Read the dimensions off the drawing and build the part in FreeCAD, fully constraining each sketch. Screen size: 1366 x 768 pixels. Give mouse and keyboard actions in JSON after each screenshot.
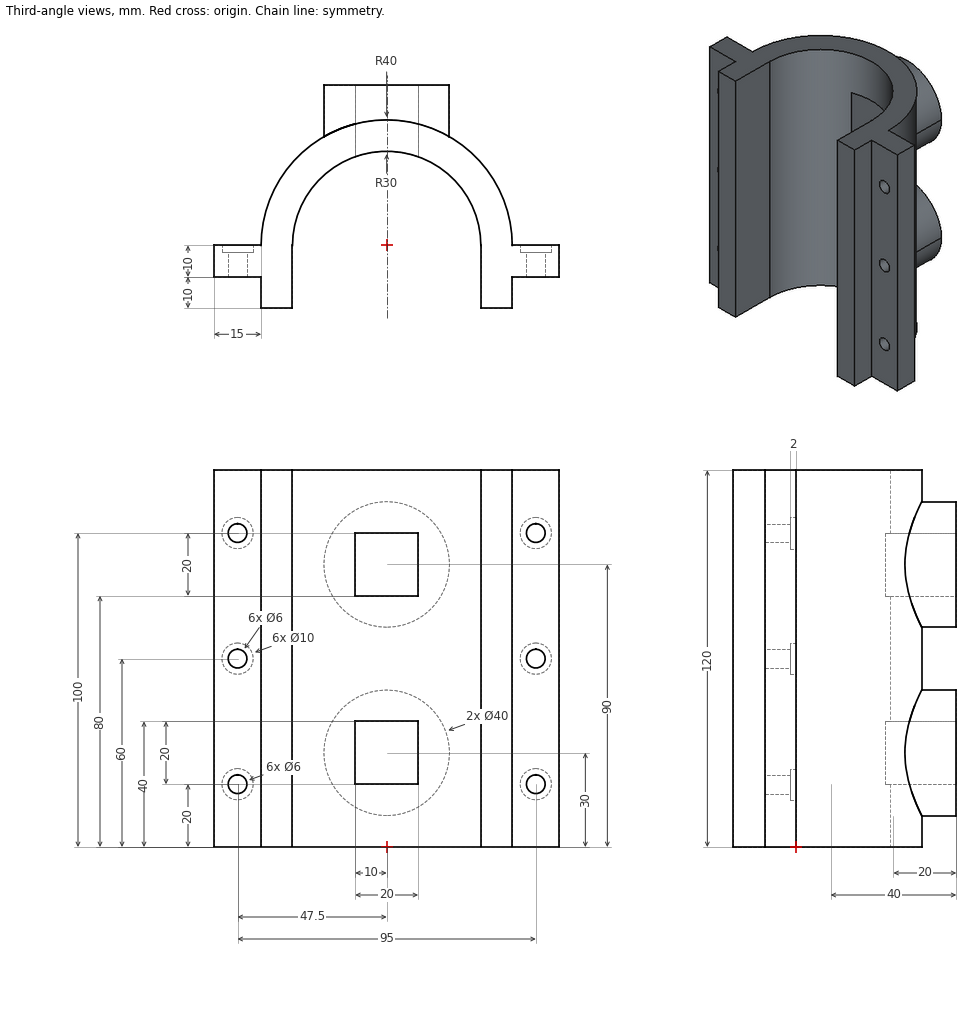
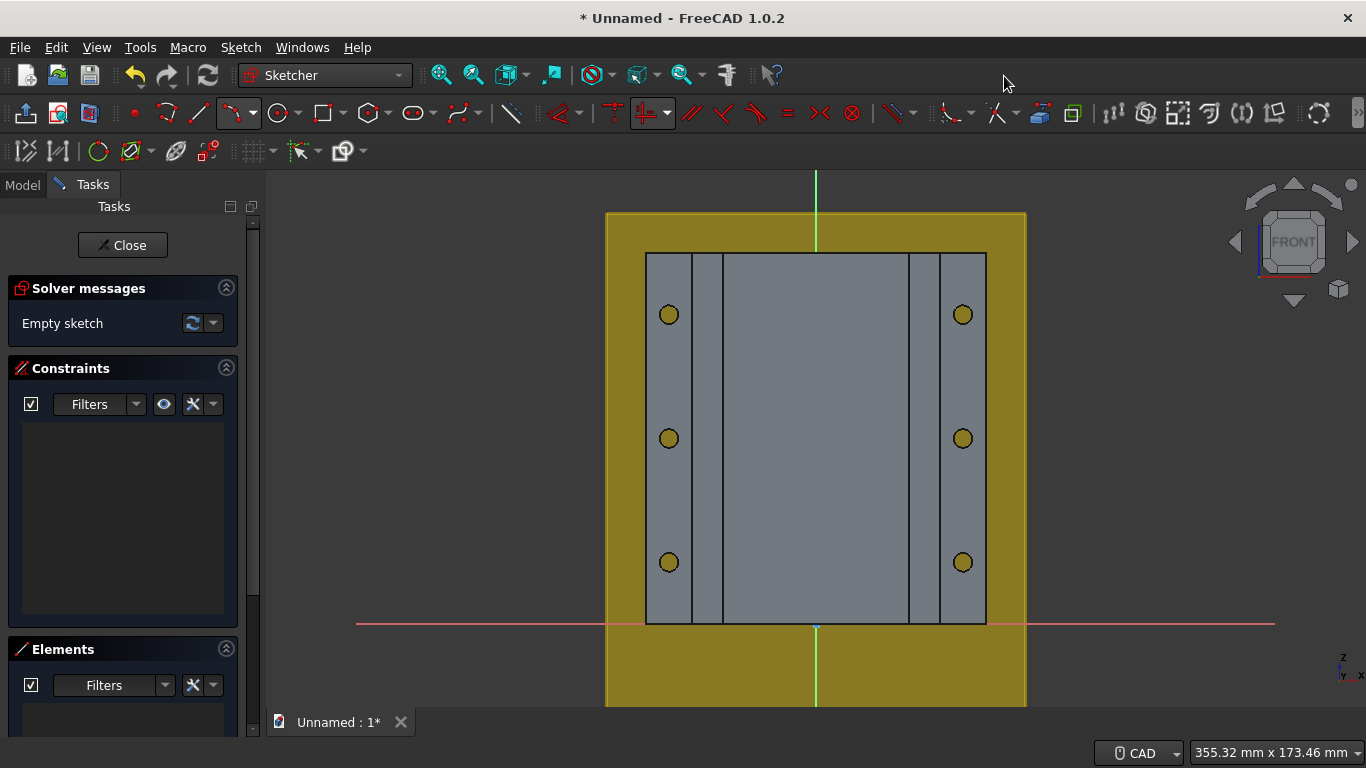
{"action": "left_click", "coordinate": [90, 114]}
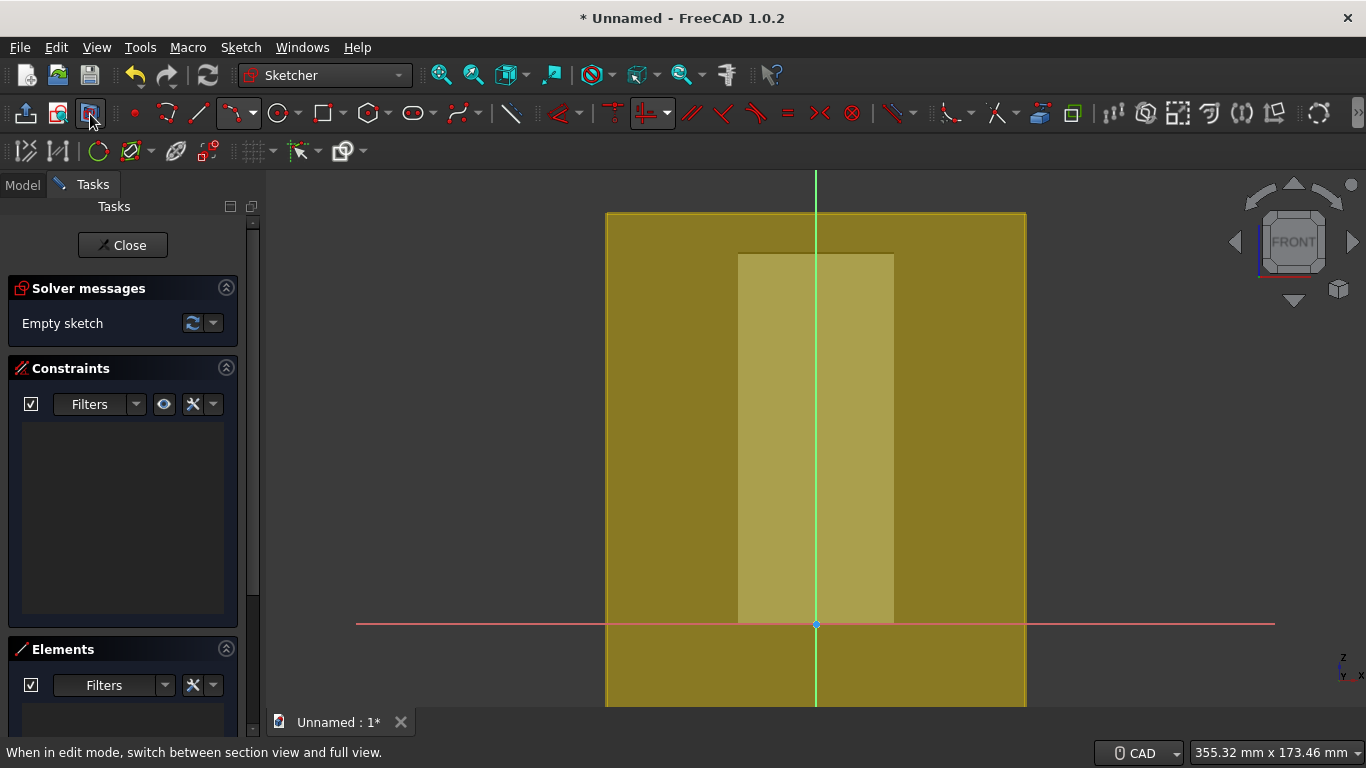
{"action": "left_click", "coordinate": [324, 114]}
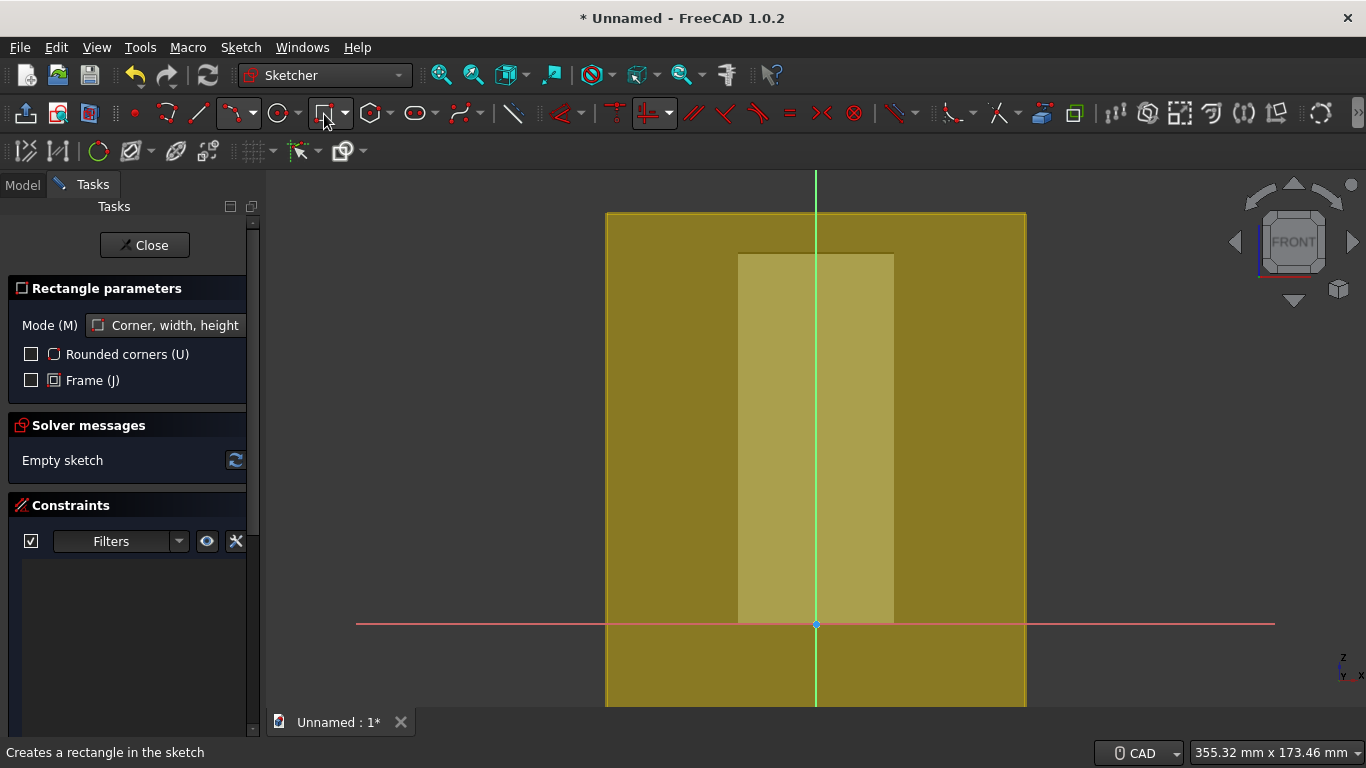
{"action": "left_click", "coordinate": [785, 500]}
{"action": "left_click", "coordinate": [847, 562]}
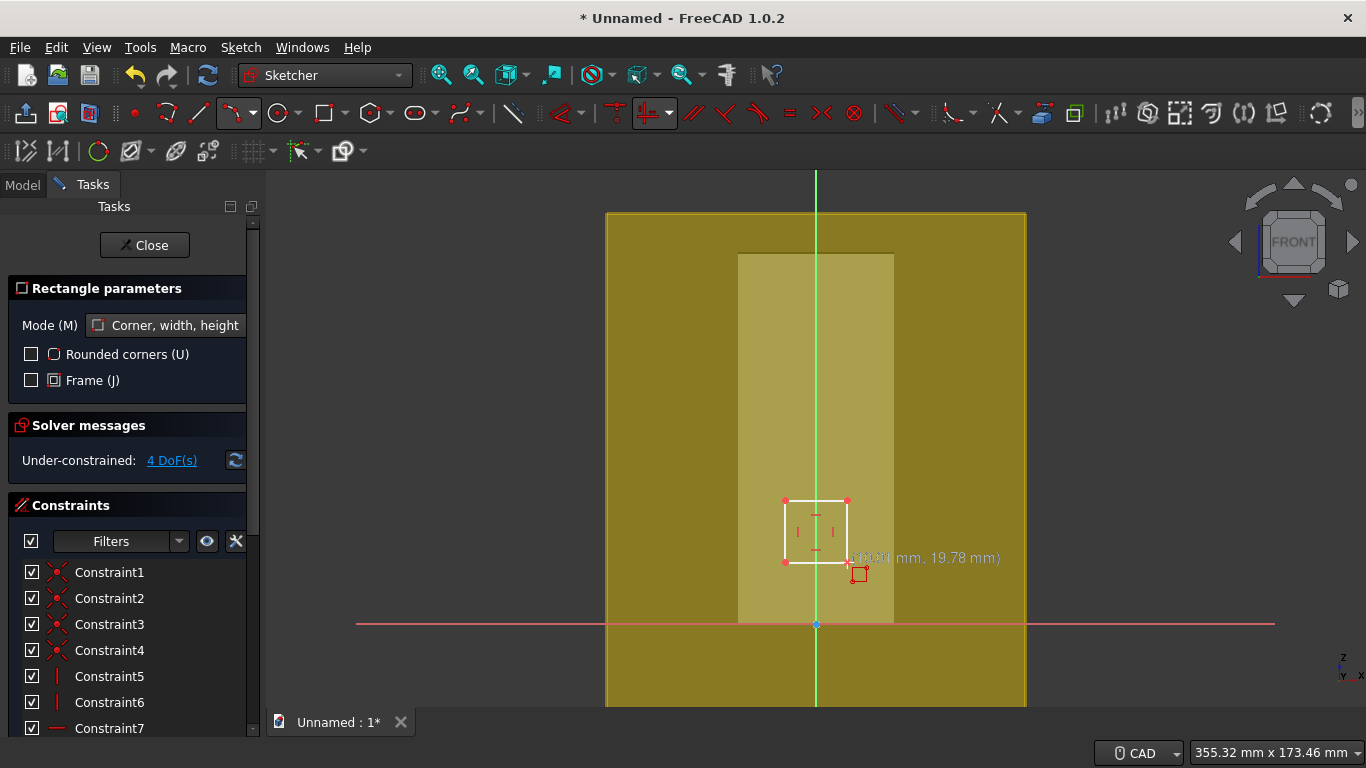
{"action": "left_click", "coordinate": [785, 315]}
{"action": "left_click", "coordinate": [847, 377]}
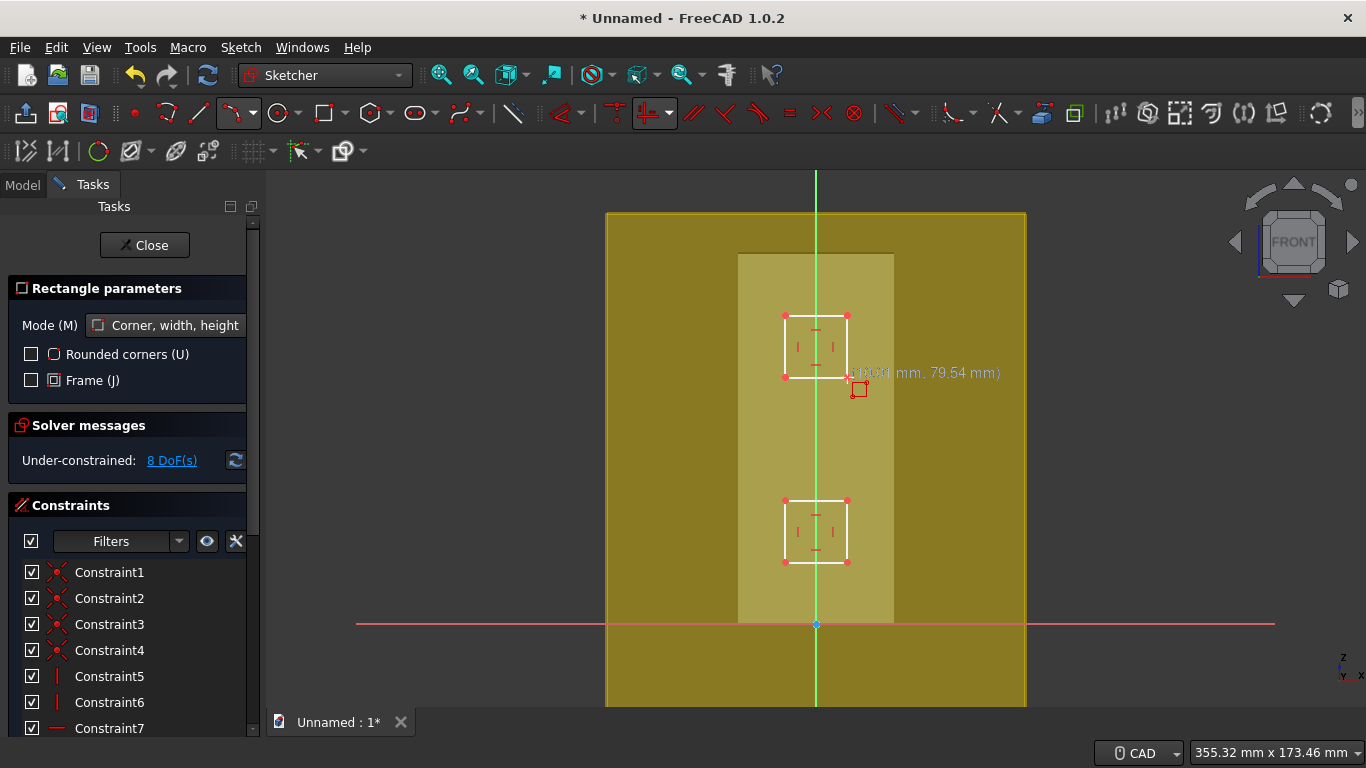
{"action": "left_click", "coordinate": [278, 114]}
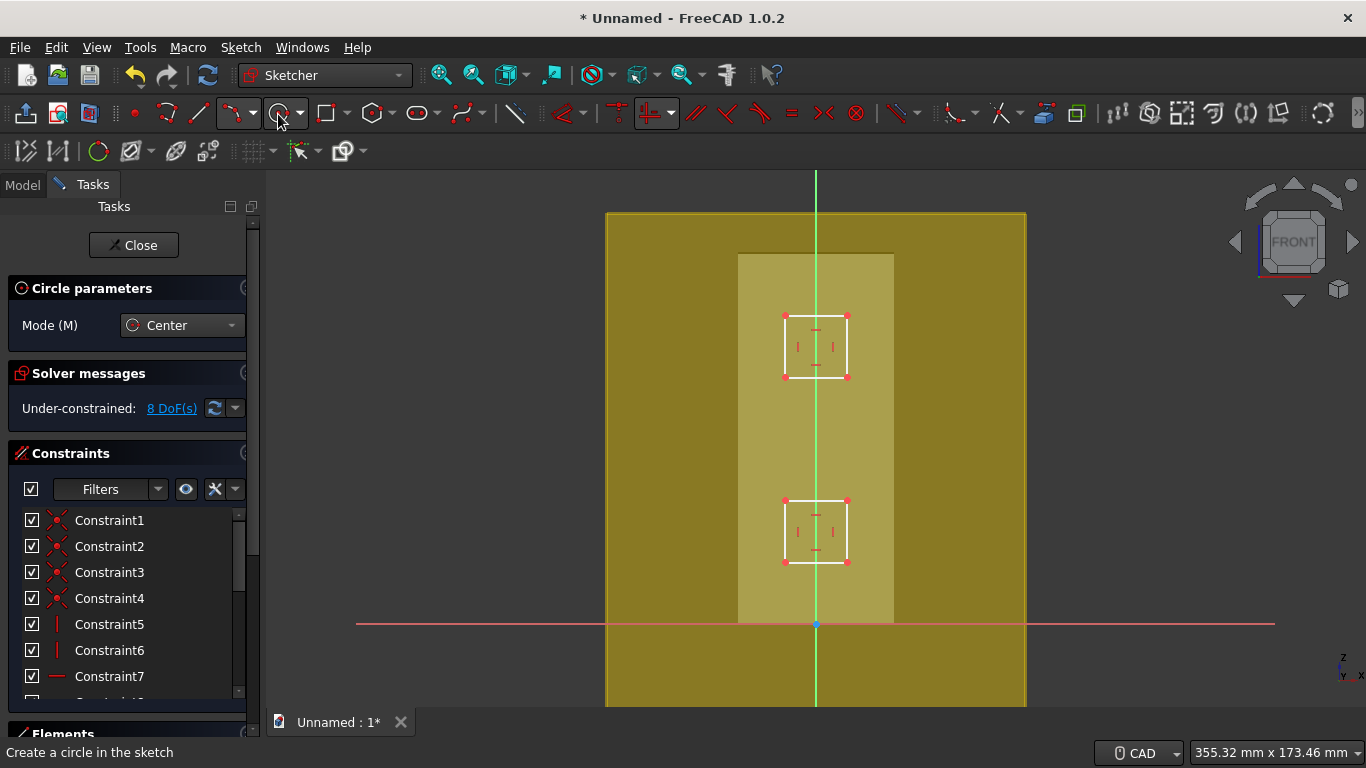
{"action": "left_click", "coordinate": [816, 531]}
{"action": "left_click", "coordinate": [860, 488]}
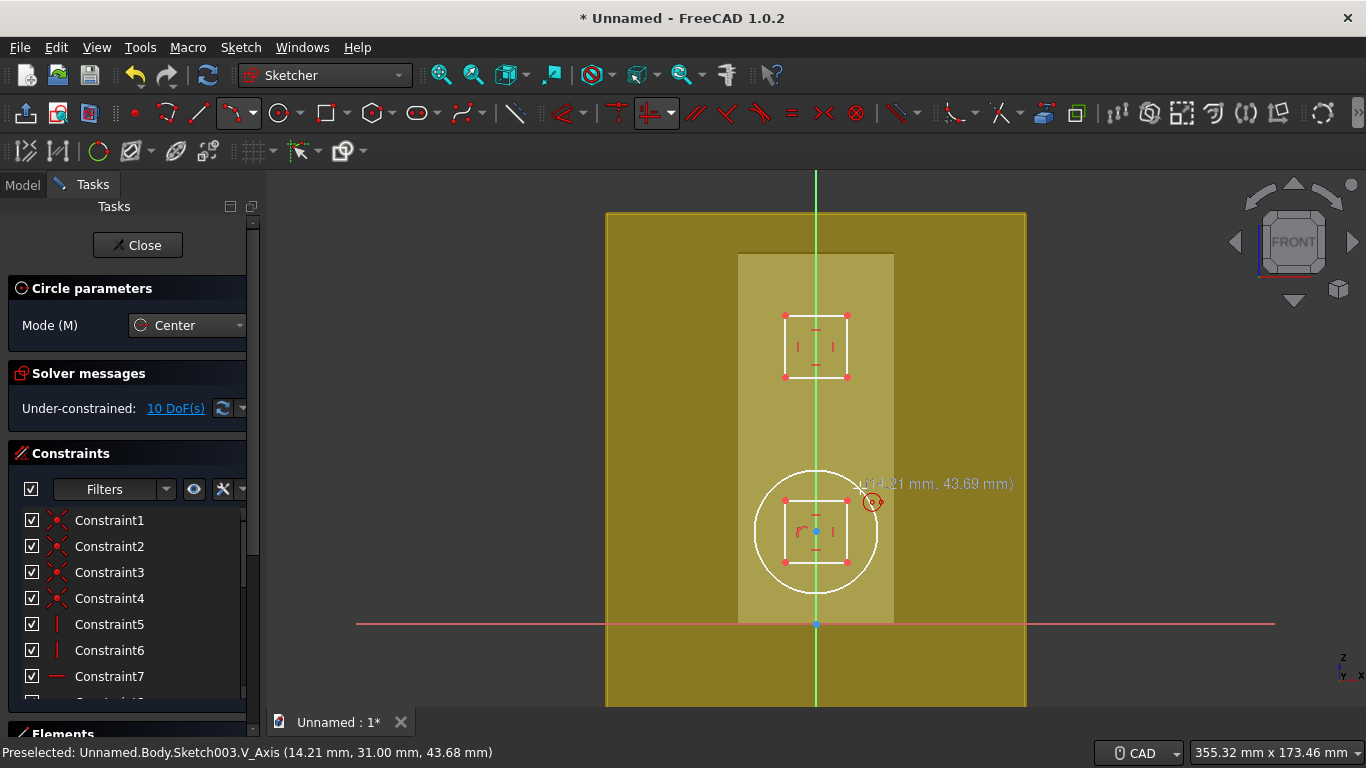
{"action": "left_click", "coordinate": [816, 346]}
{"action": "left_click", "coordinate": [860, 302]}
{"action": "key", "text": "Escape"}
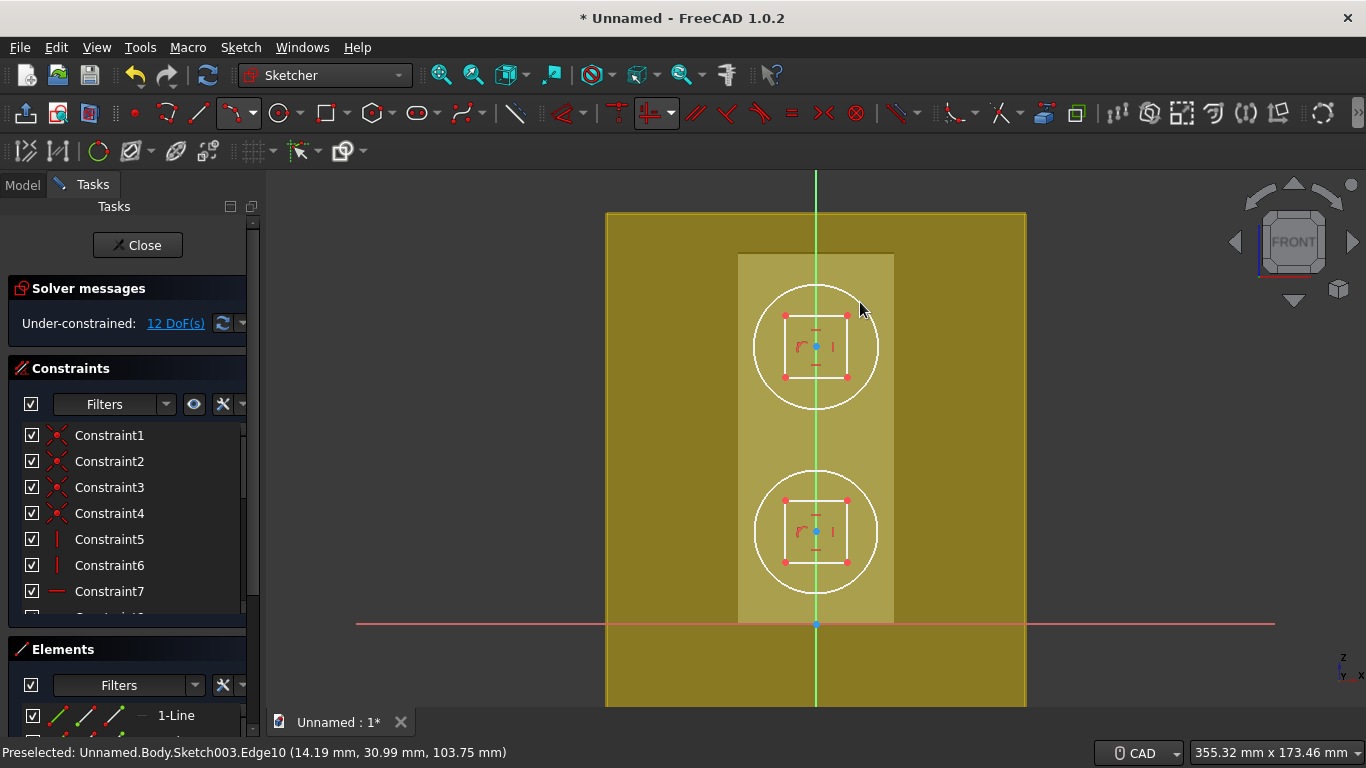
{"action": "left_click", "coordinate": [859, 488]}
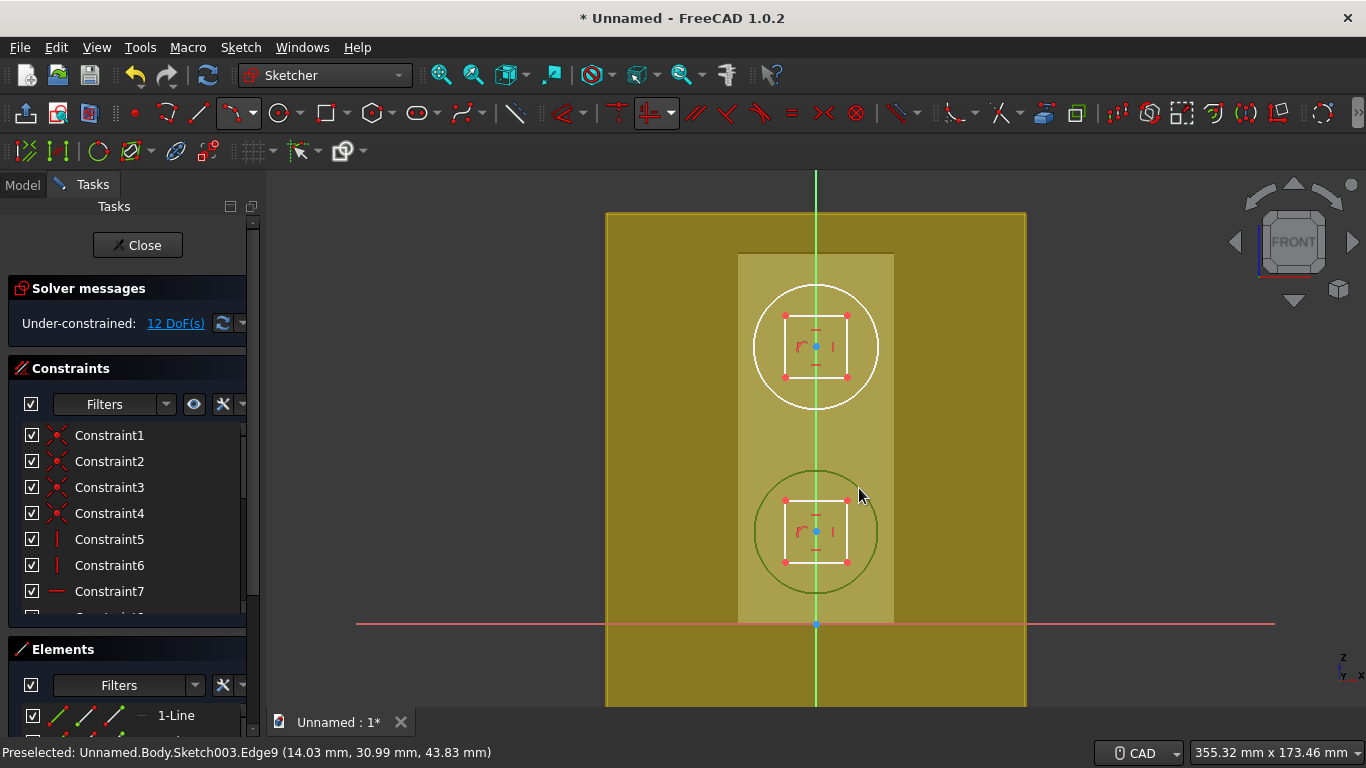
{"action": "left_click", "coordinate": [860, 303]}